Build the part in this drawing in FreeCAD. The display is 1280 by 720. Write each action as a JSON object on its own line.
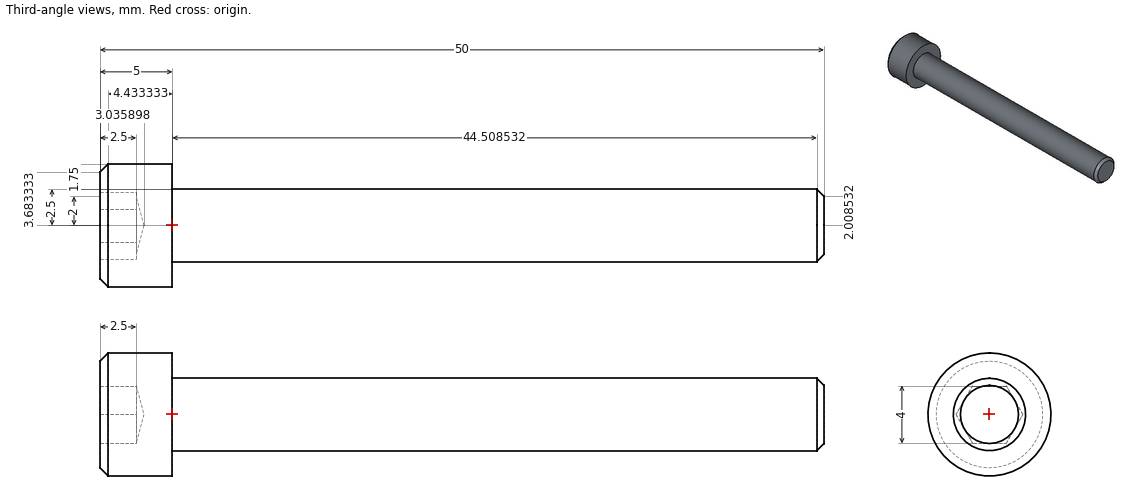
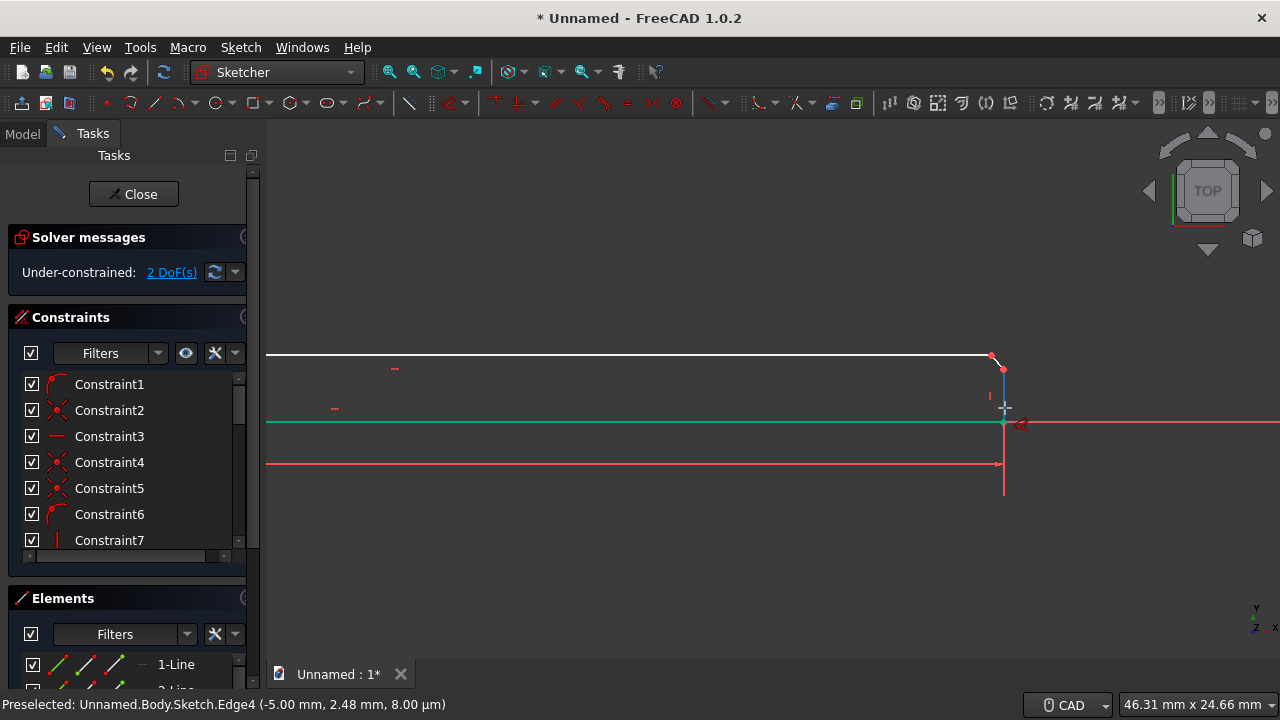
{"action": "left_click", "coordinate": [1004, 406]}
{"action": "left_click", "coordinate": [1038, 396]}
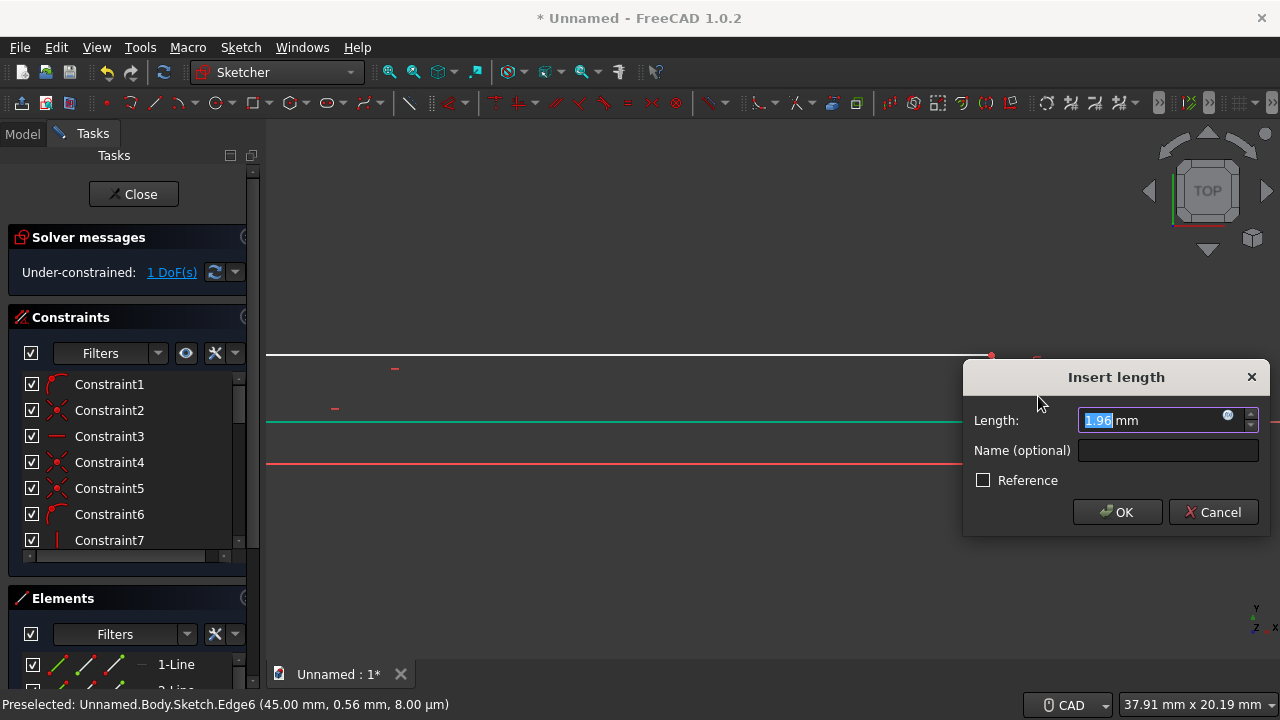
{"action": "type", "text": "2.008532"}
{"action": "key", "text": "Return"}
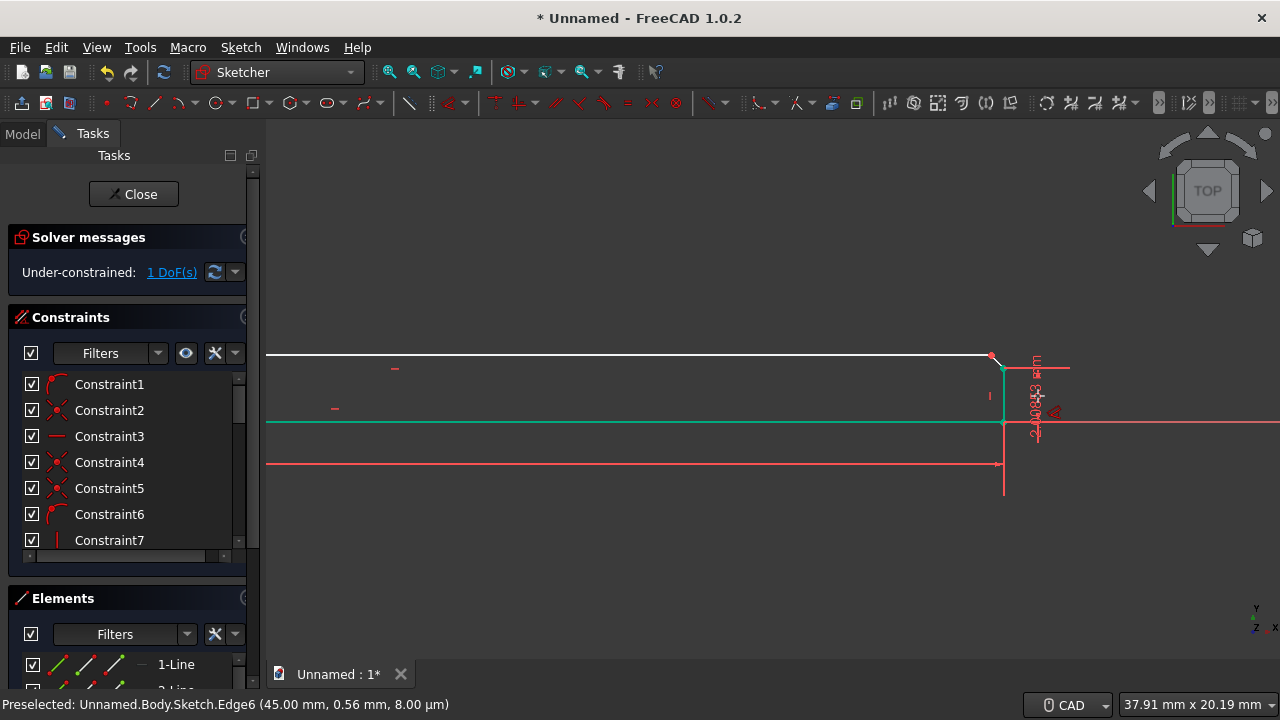
{"action": "left_click", "coordinate": [634, 355]}
{"action": "left_click", "coordinate": [643, 321]}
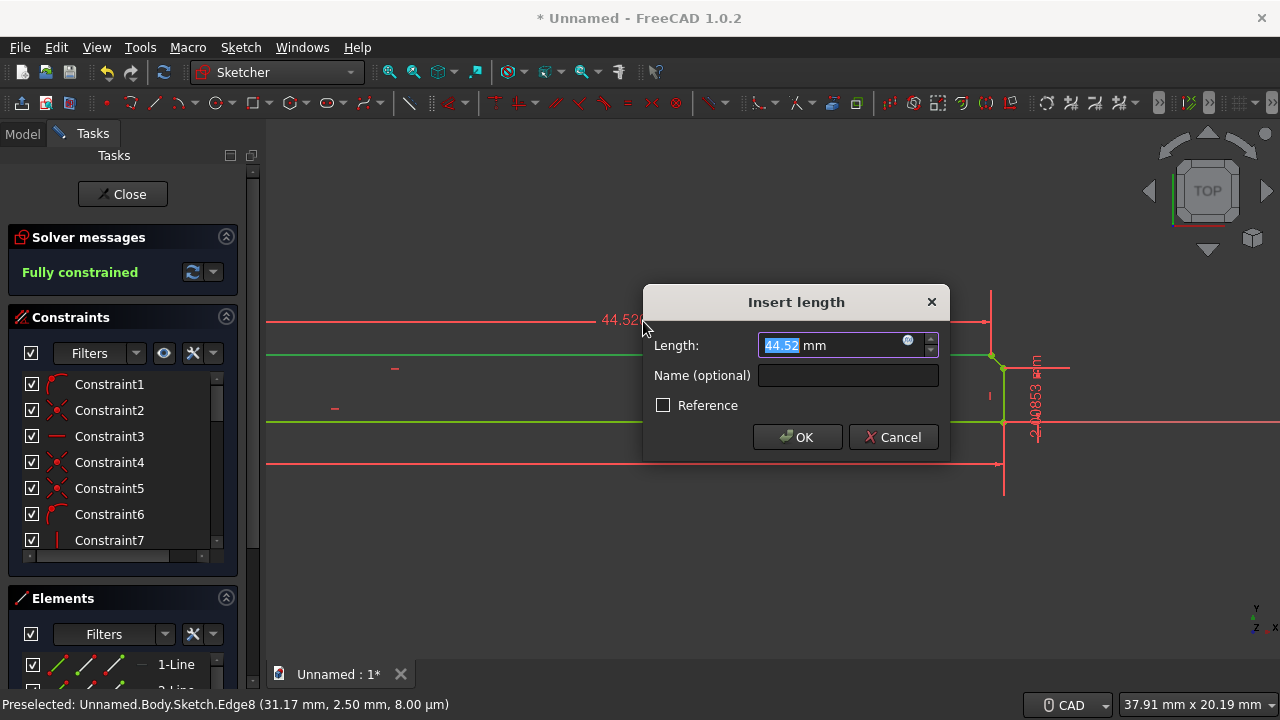
{"action": "type", "text": "44.508532"}
{"action": "key", "text": "Return"}
{"action": "key", "text": "Escape"}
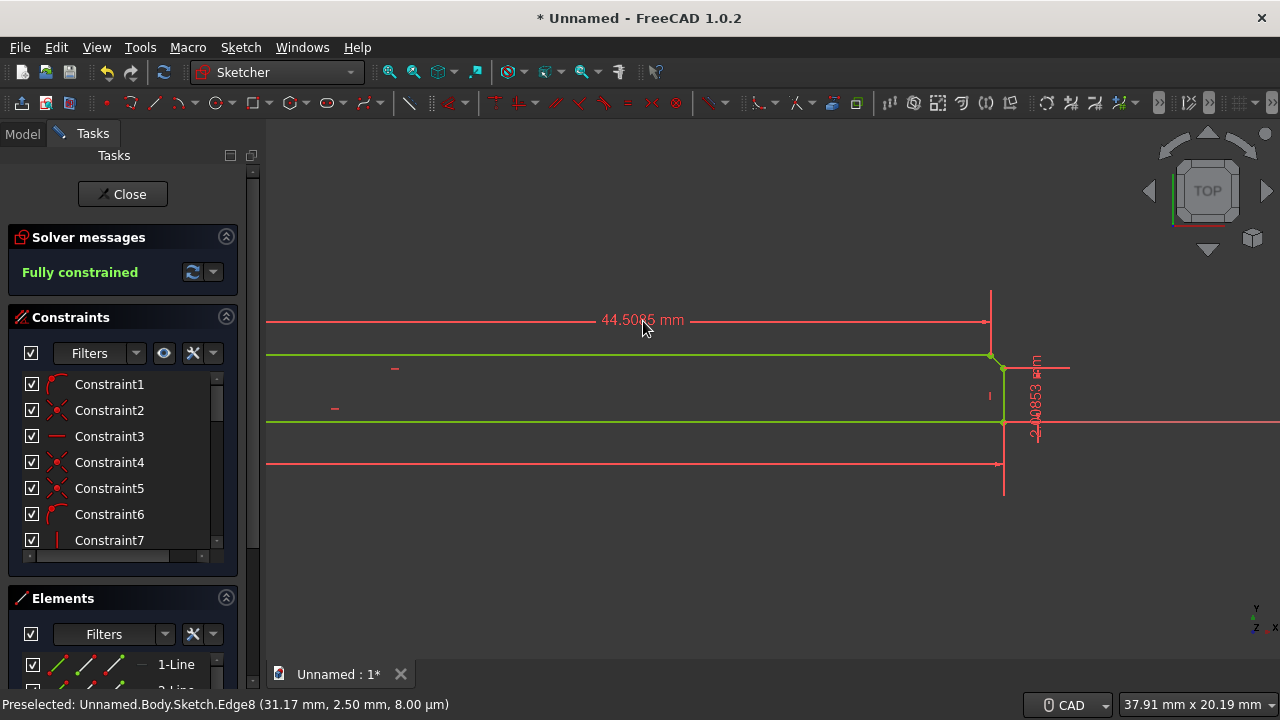
{"action": "left_click", "coordinate": [123, 194]}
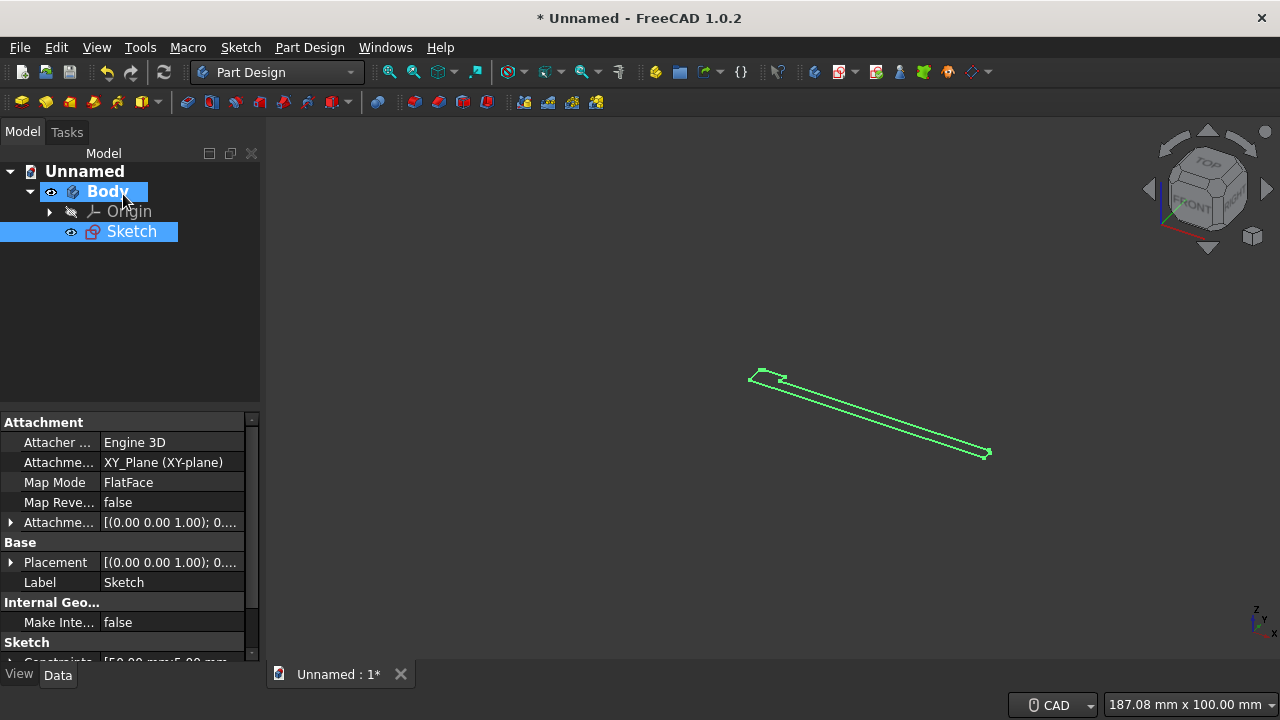
{"action": "left_click", "coordinate": [46, 102]}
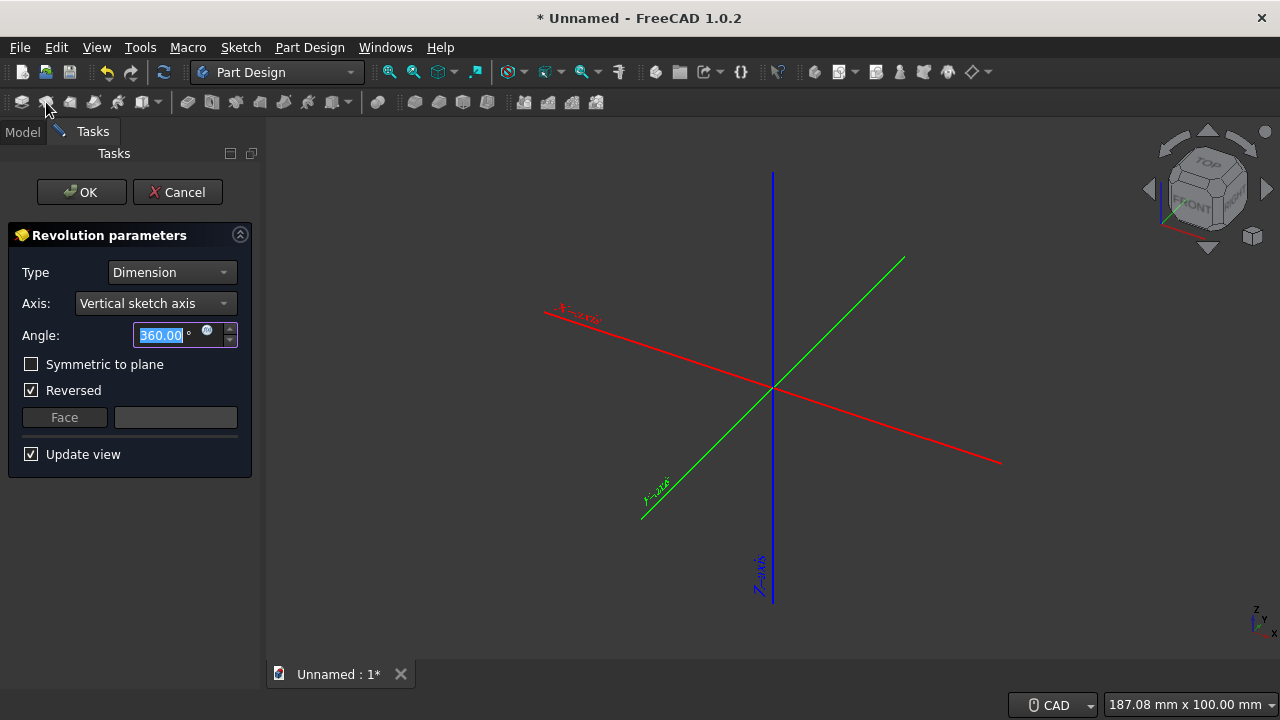
{"action": "left_click", "coordinate": [156, 304]}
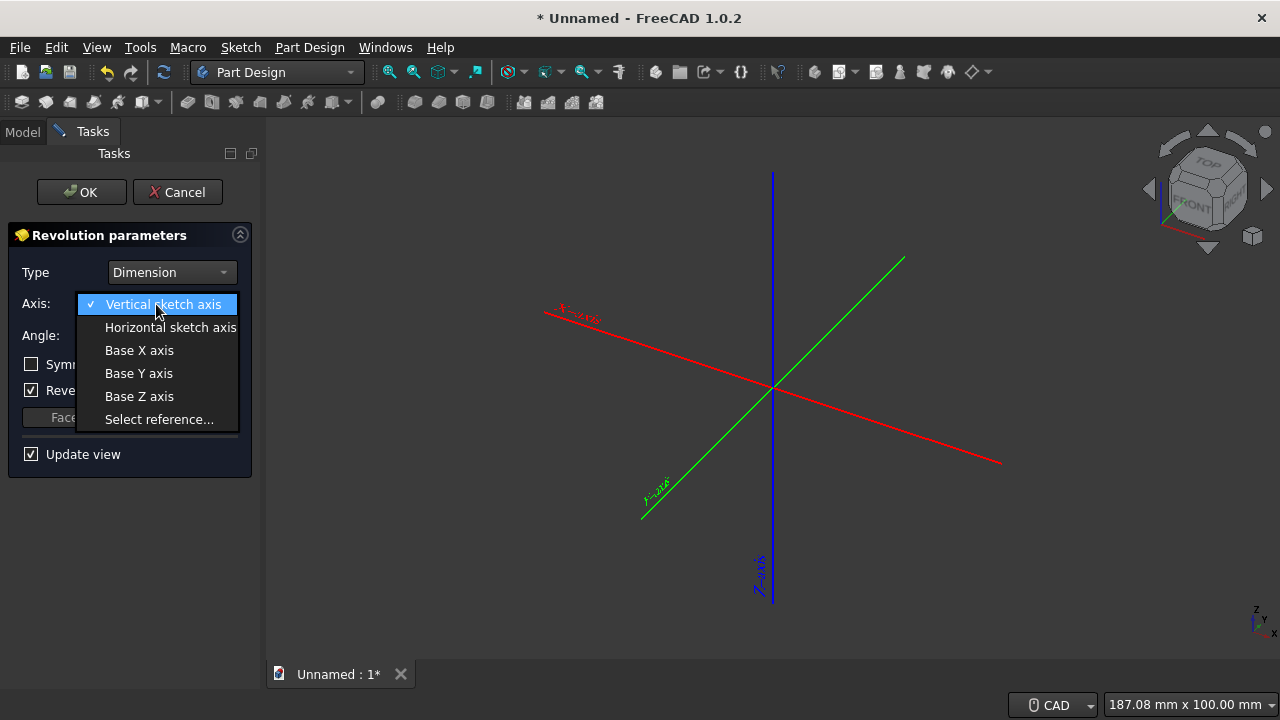
{"action": "left_click", "coordinate": [156, 328]}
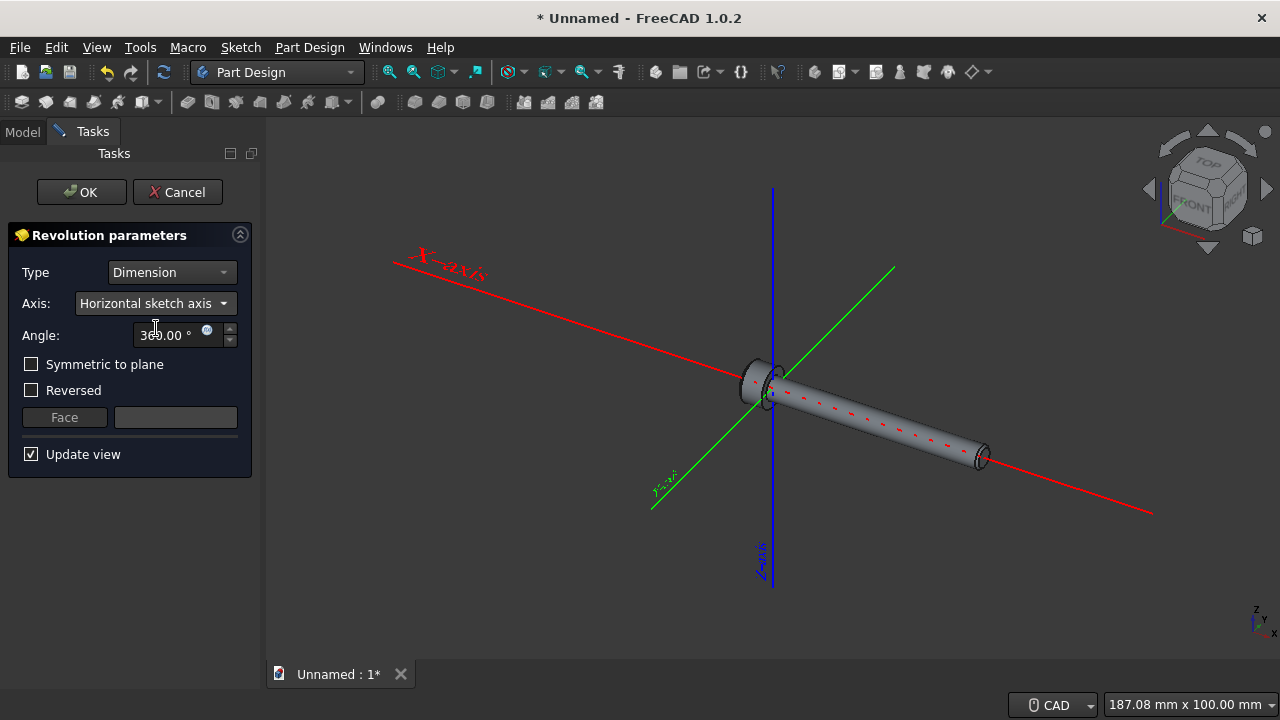
{"action": "left_click", "coordinate": [82, 192]}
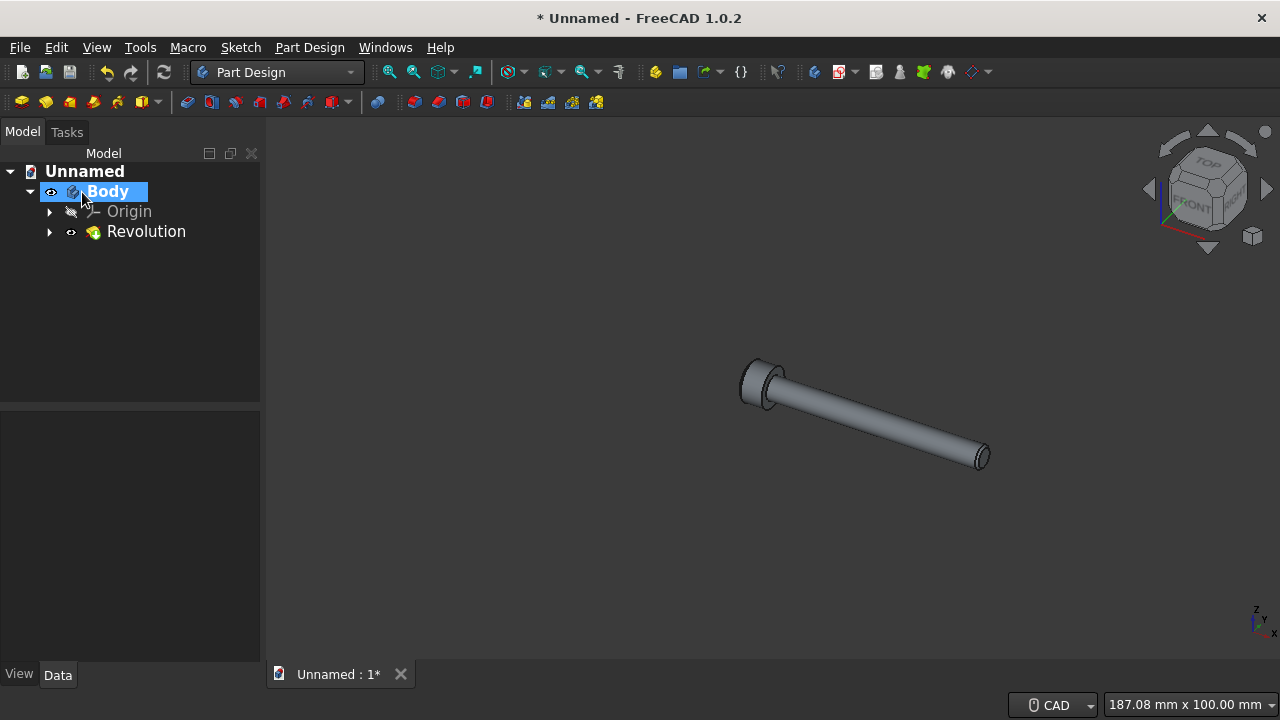
{"action": "left_click", "coordinate": [390, 72]}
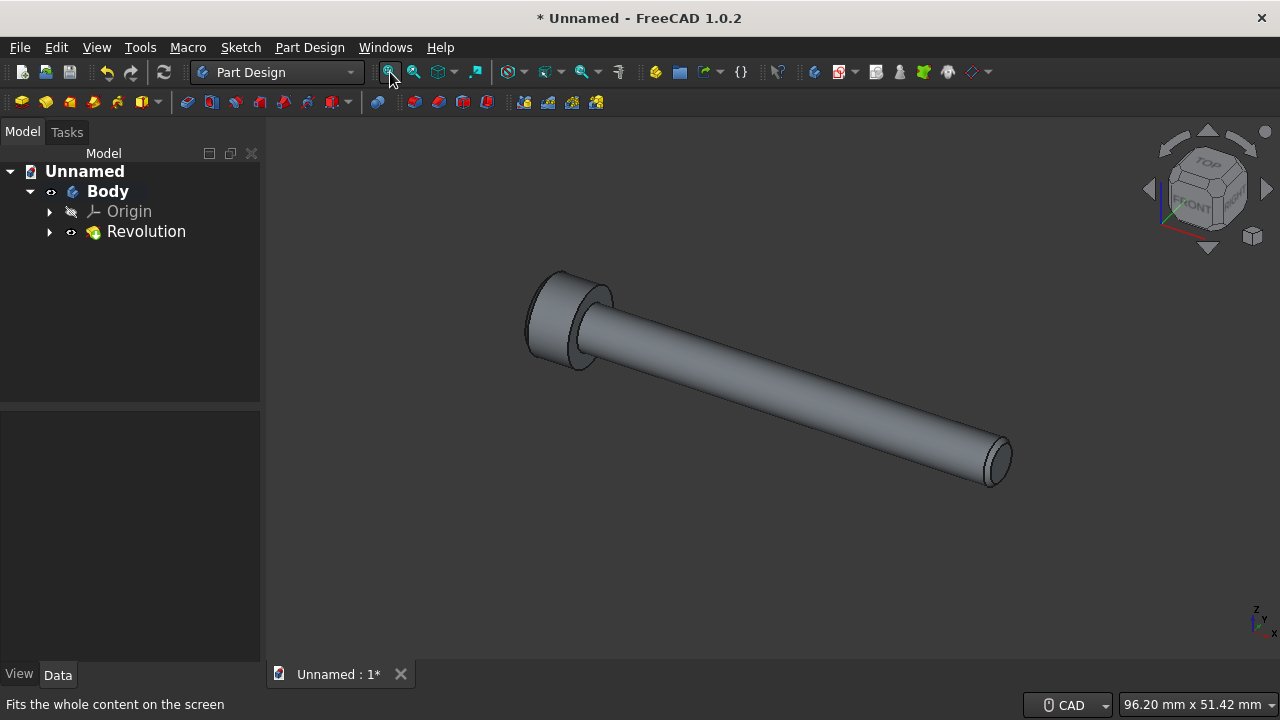
{"action": "left_click", "coordinate": [840, 72]}